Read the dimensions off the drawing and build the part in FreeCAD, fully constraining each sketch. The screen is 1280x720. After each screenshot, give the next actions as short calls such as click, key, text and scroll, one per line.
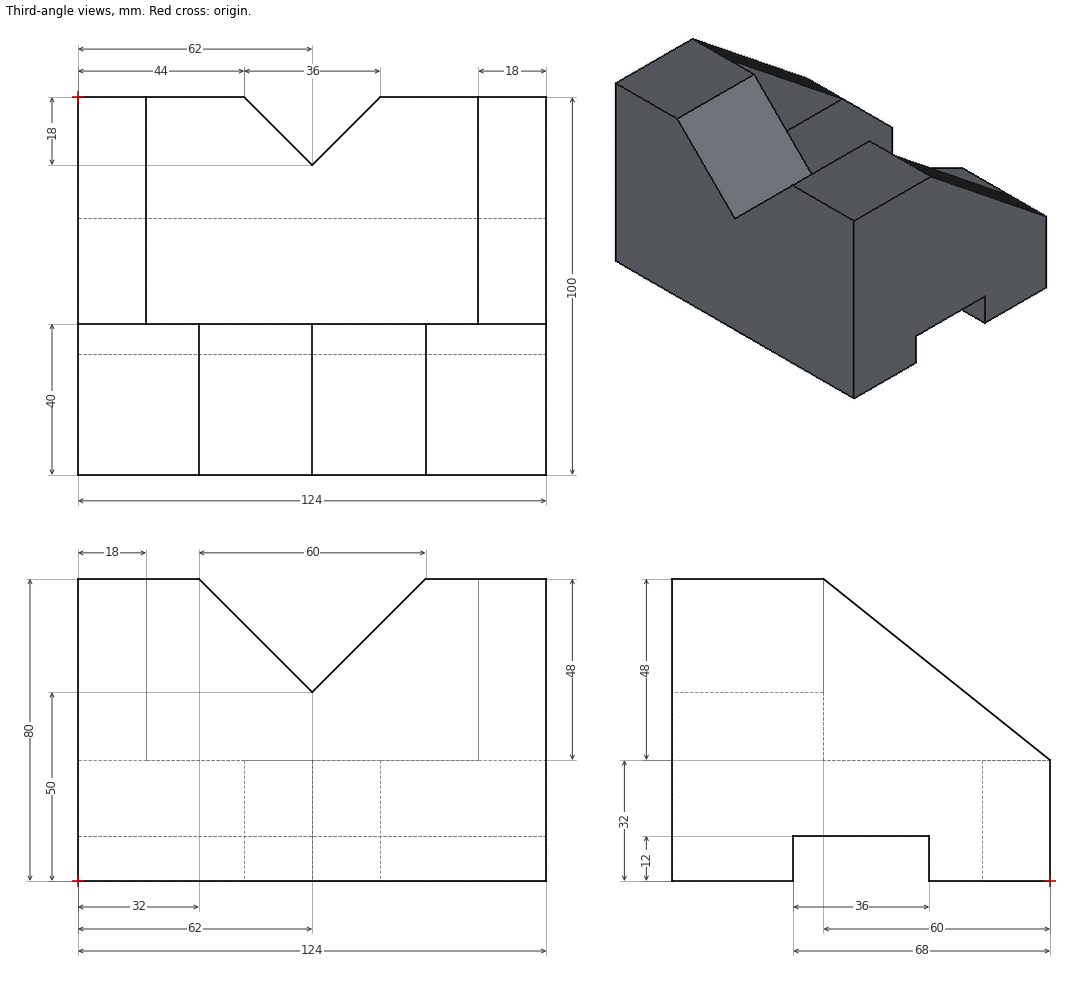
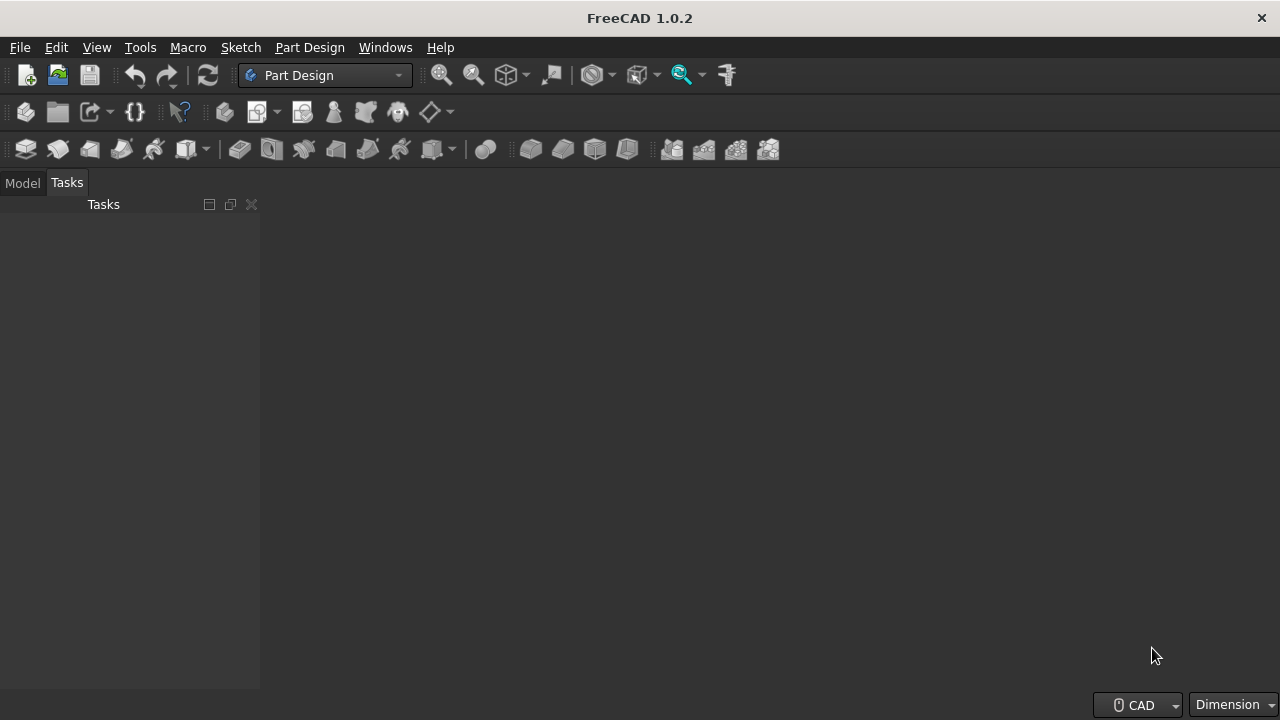
click(26, 76)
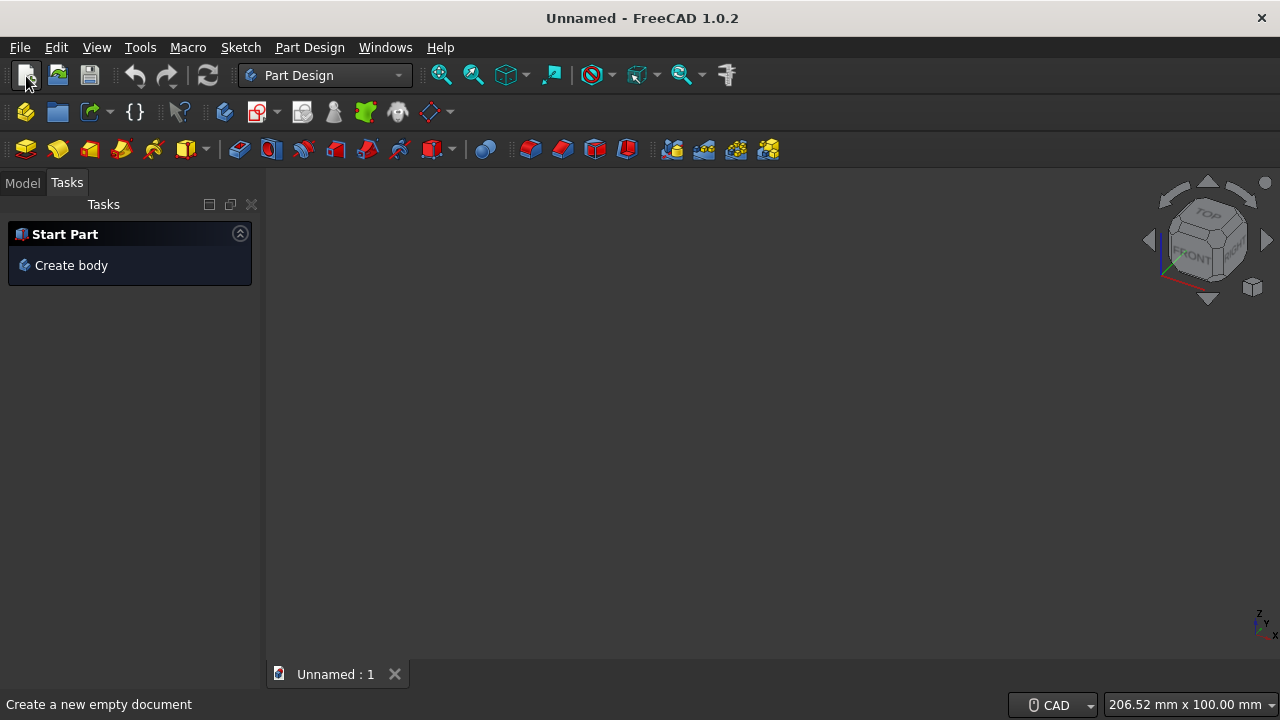
click(258, 112)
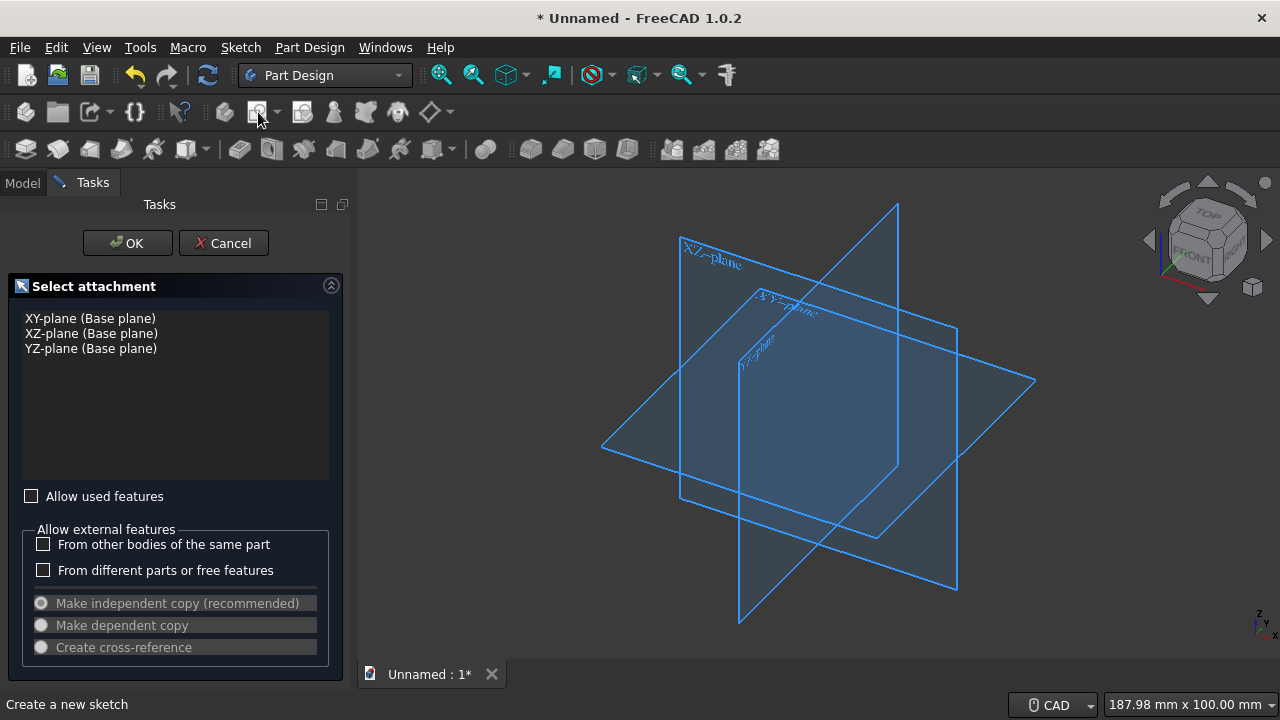
click(82, 318)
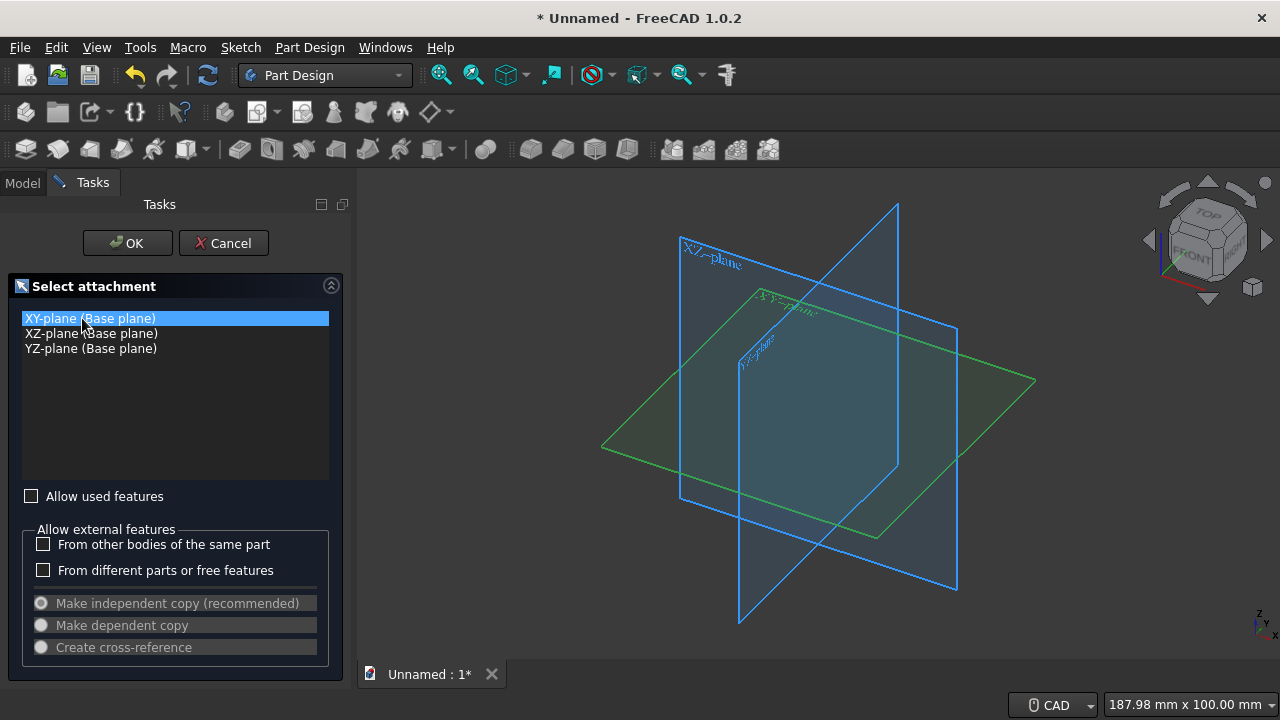
click(128, 243)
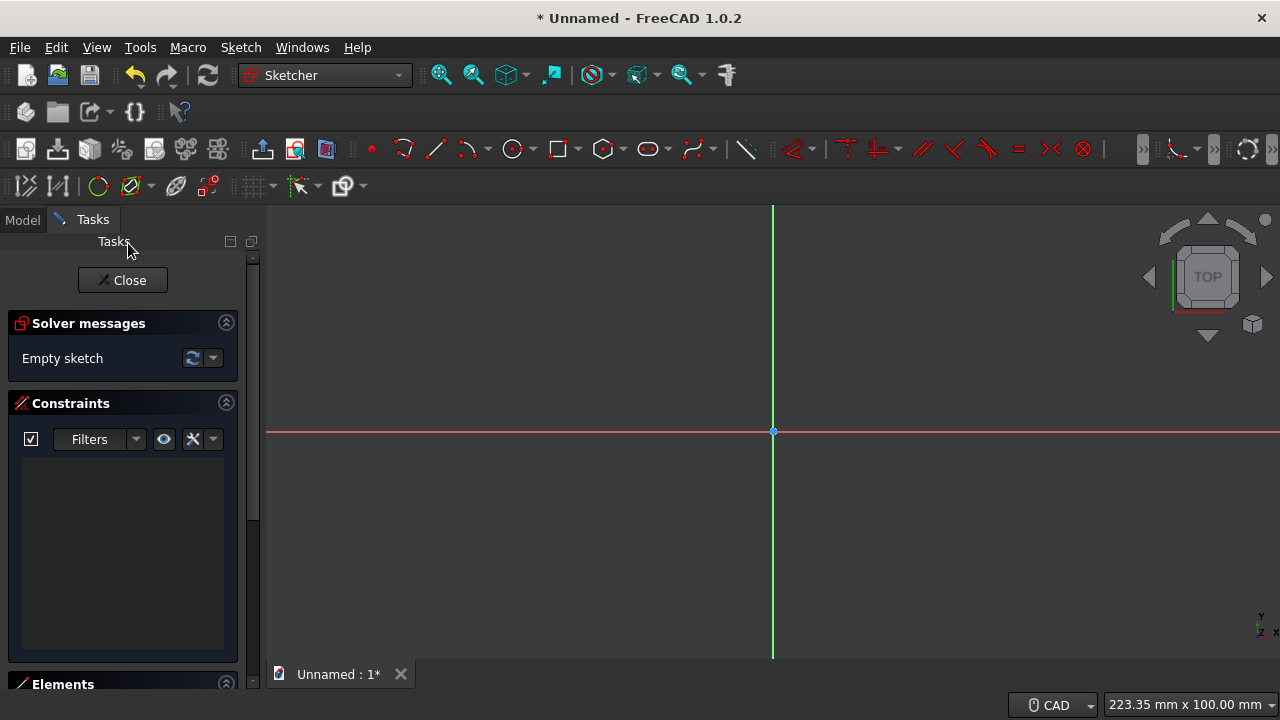
scroll(294, 233, down, 3)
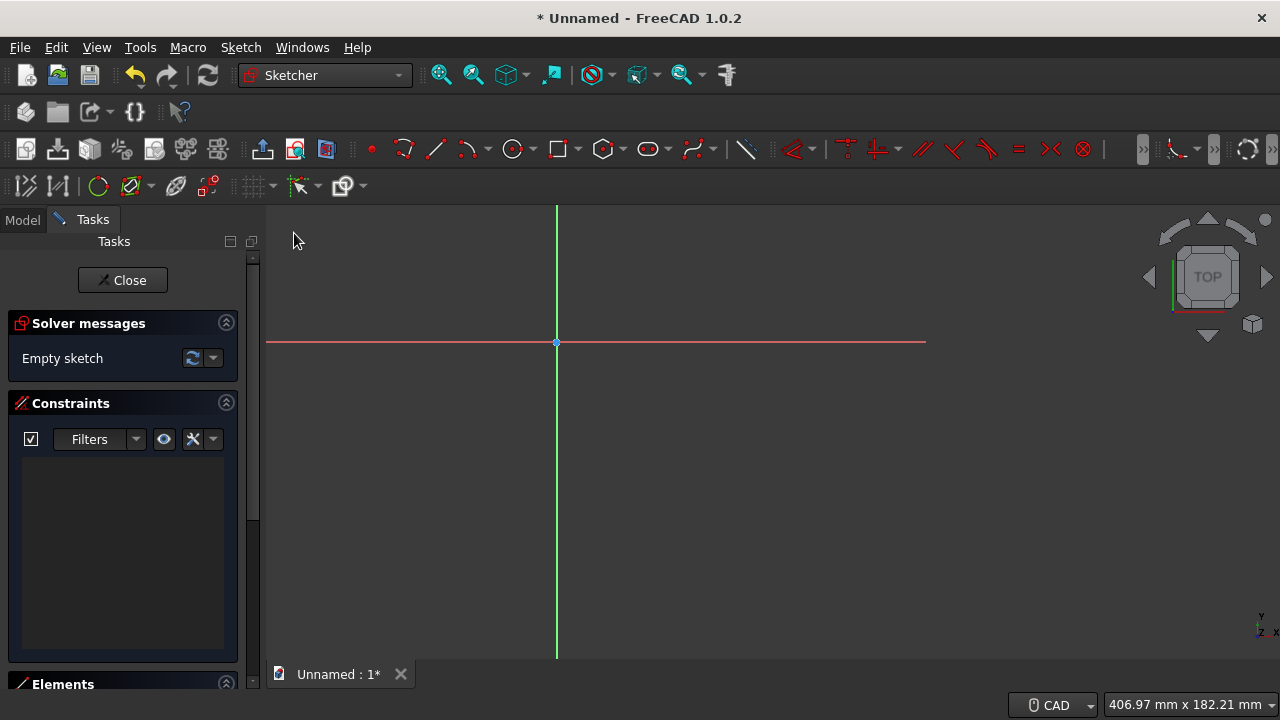
click(558, 150)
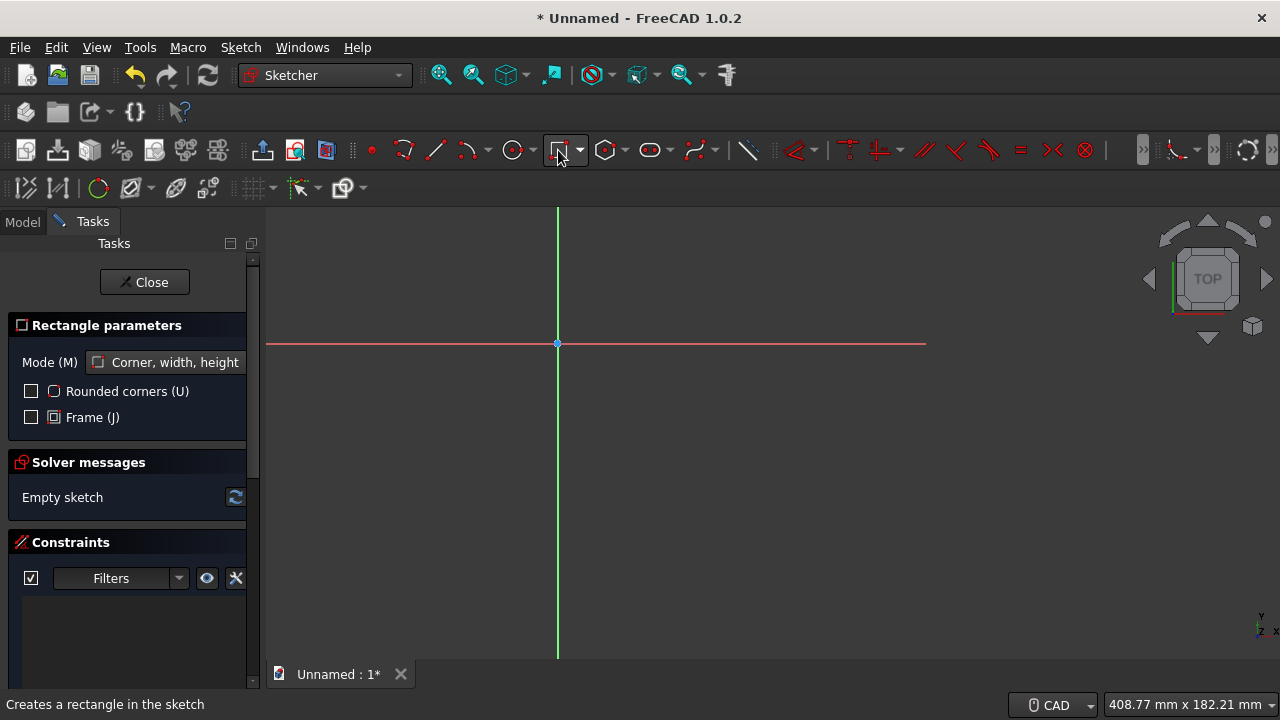
click(558, 344)
move(865, 592)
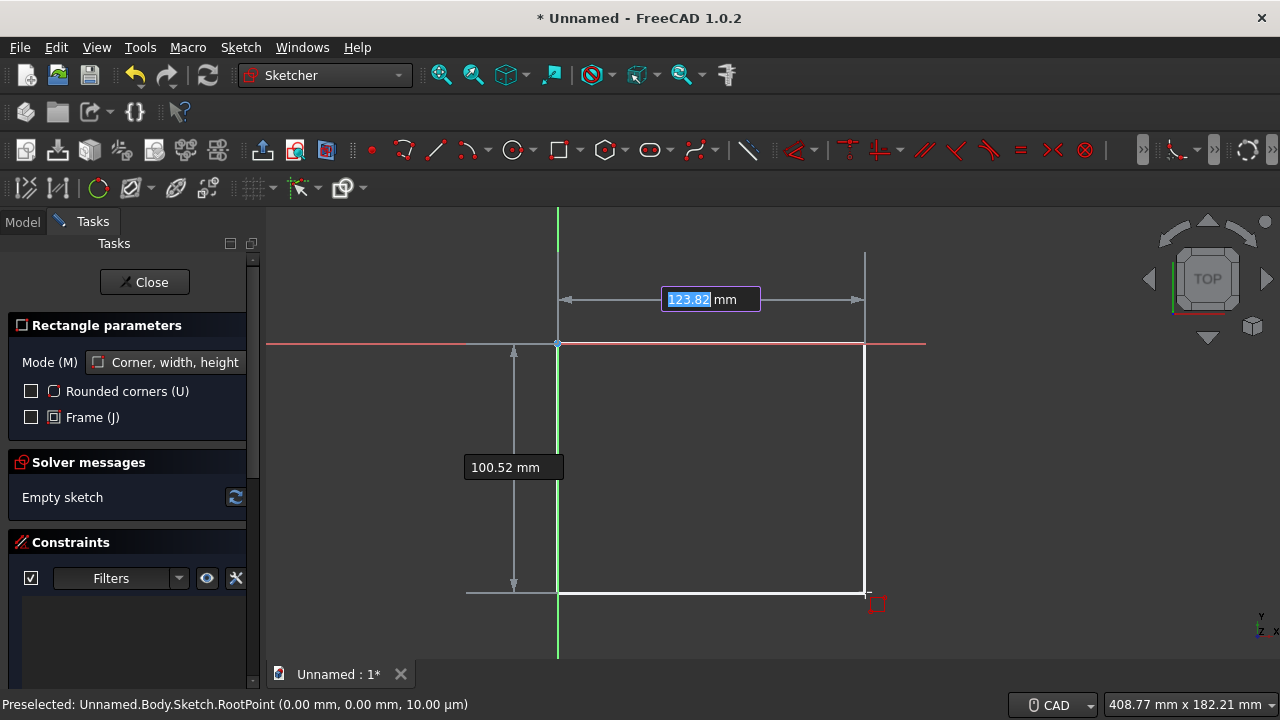
text(124)
key(Tab)
text(100)
key(Return)
key(Escape)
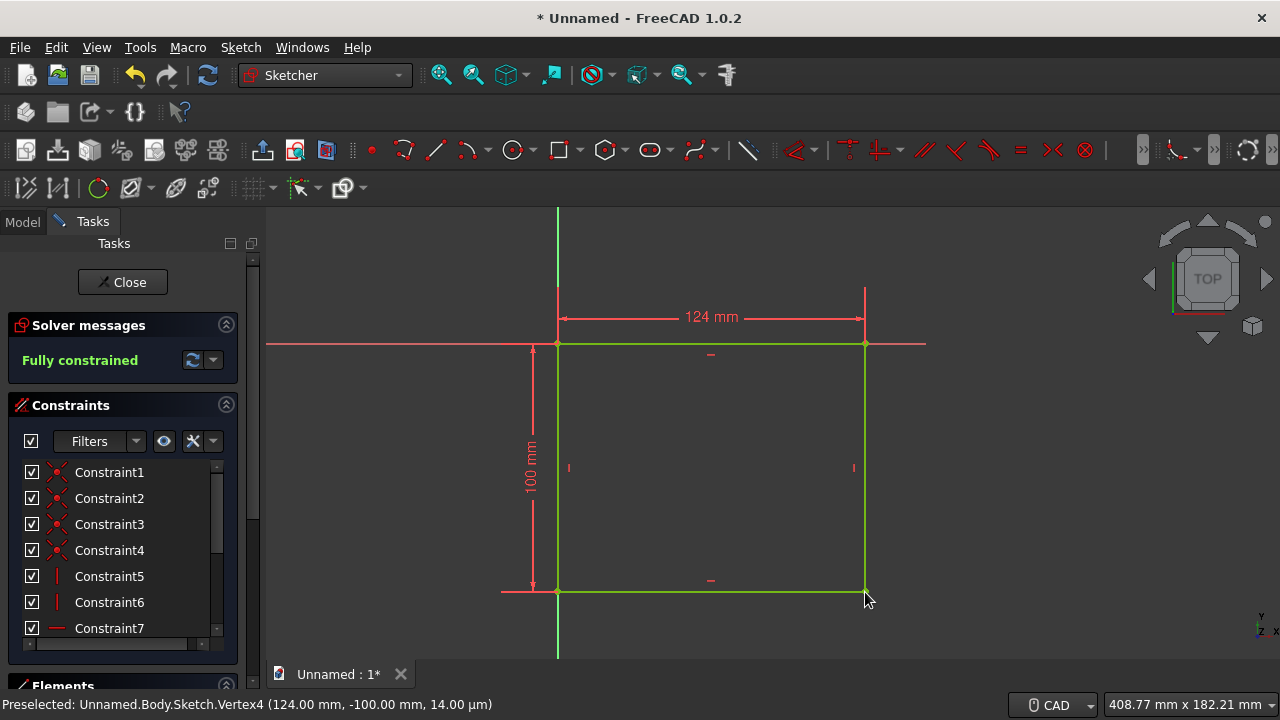
click(123, 282)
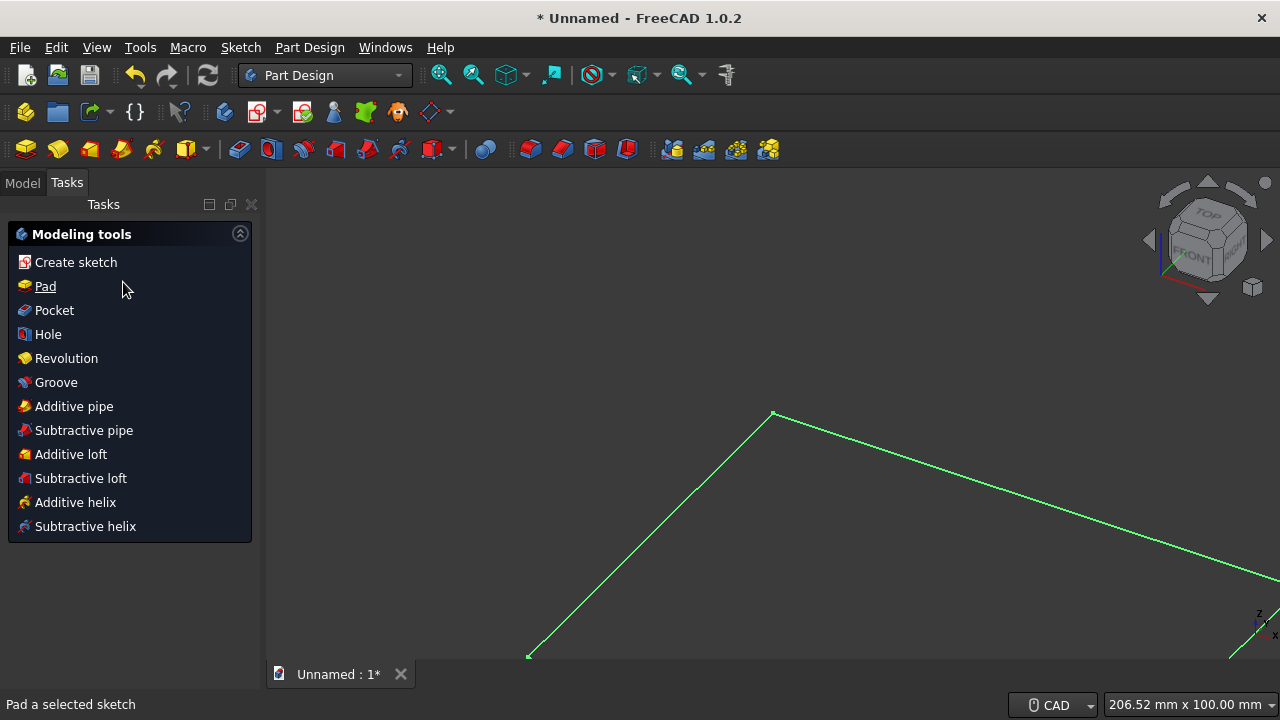
click(26, 150)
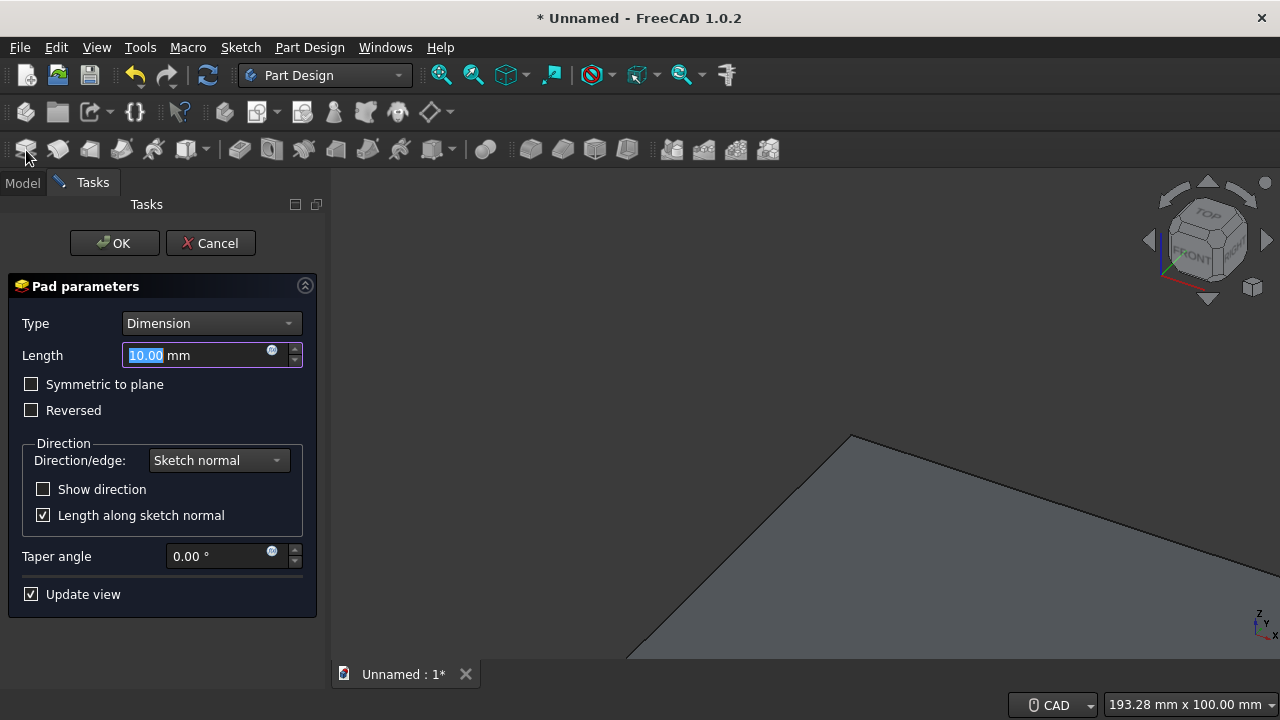
text(32)
key(Tab)